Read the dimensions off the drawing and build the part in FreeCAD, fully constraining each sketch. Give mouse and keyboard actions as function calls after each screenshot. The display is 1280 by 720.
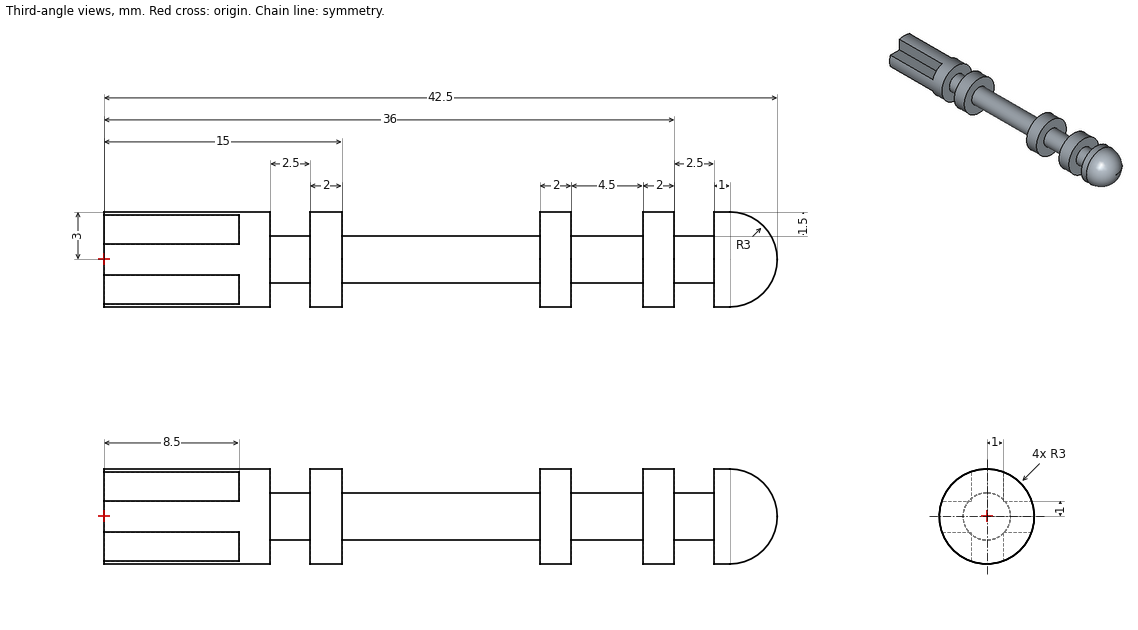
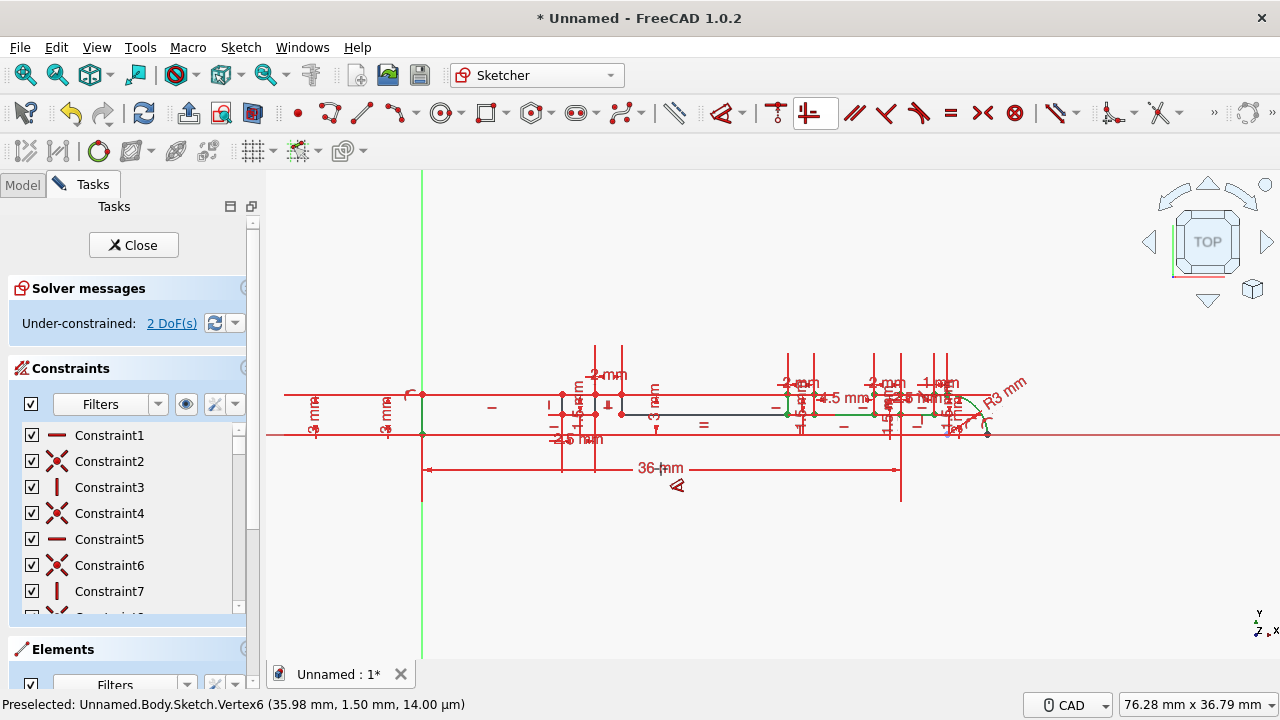
click(622, 415)
click(522, 469)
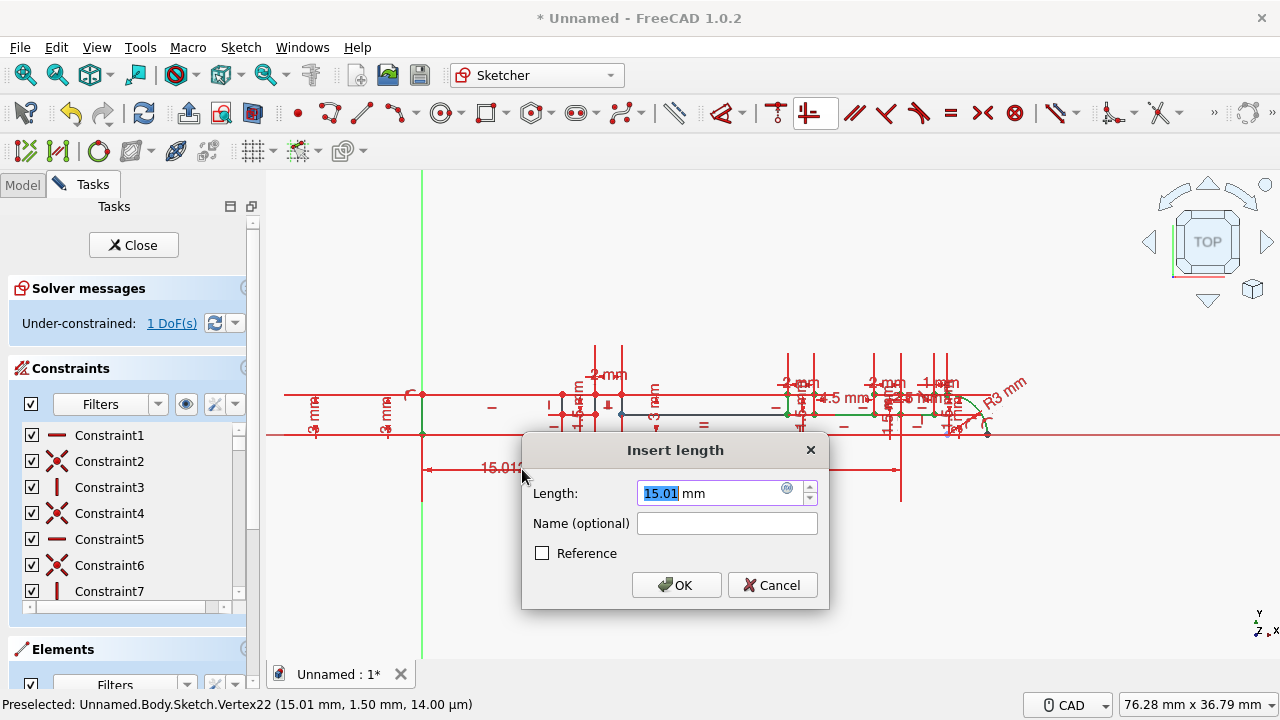
text(15)
key(Return)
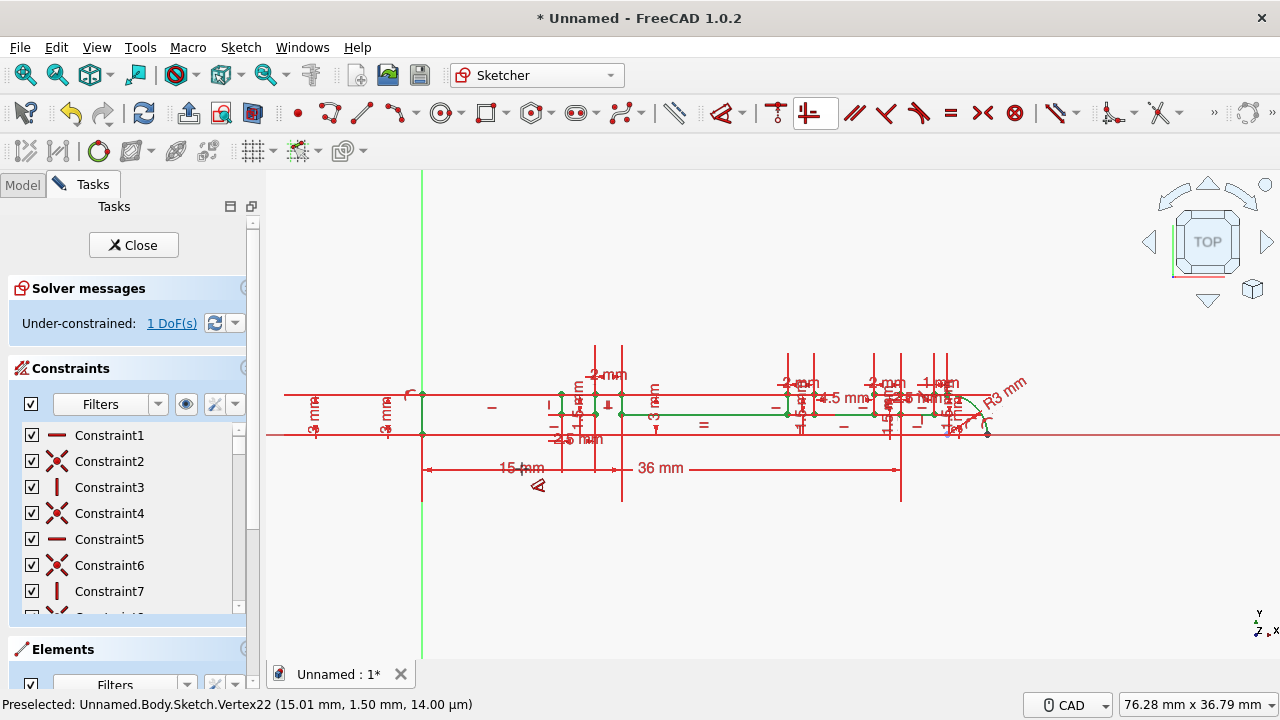
click(592, 435)
click(835, 469)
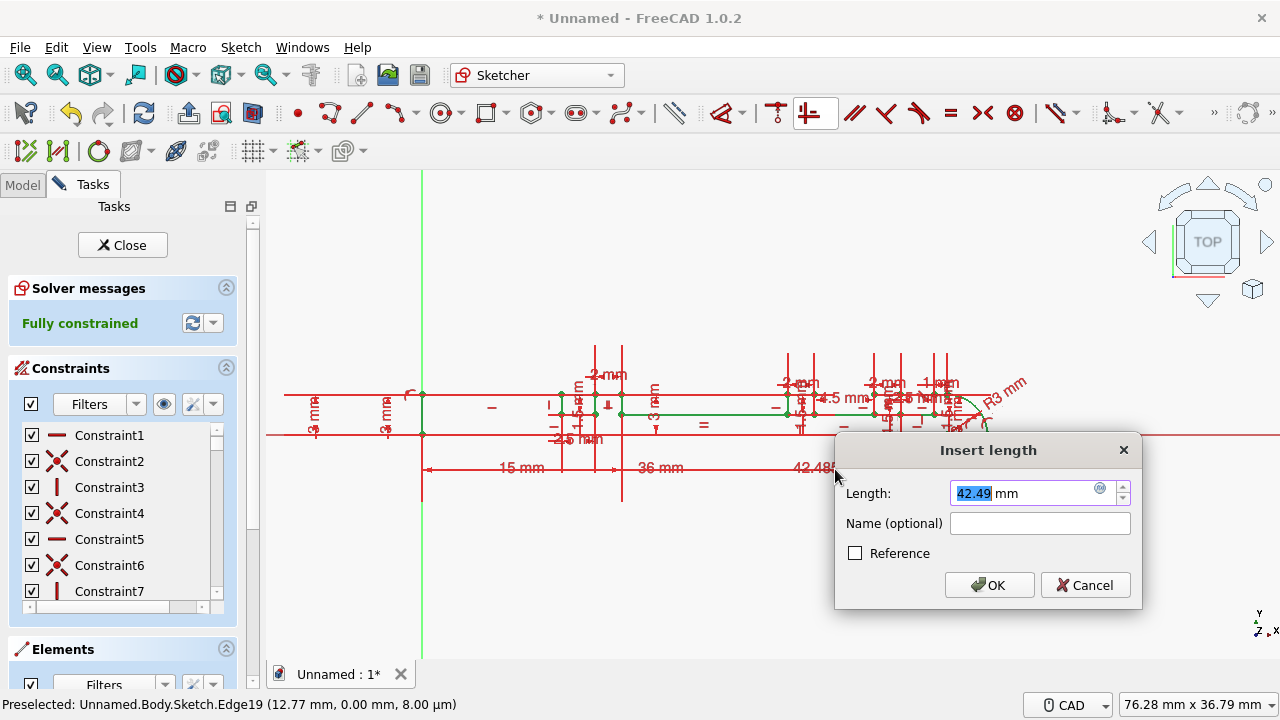
text(42.5)
key(Return)
key(Escape)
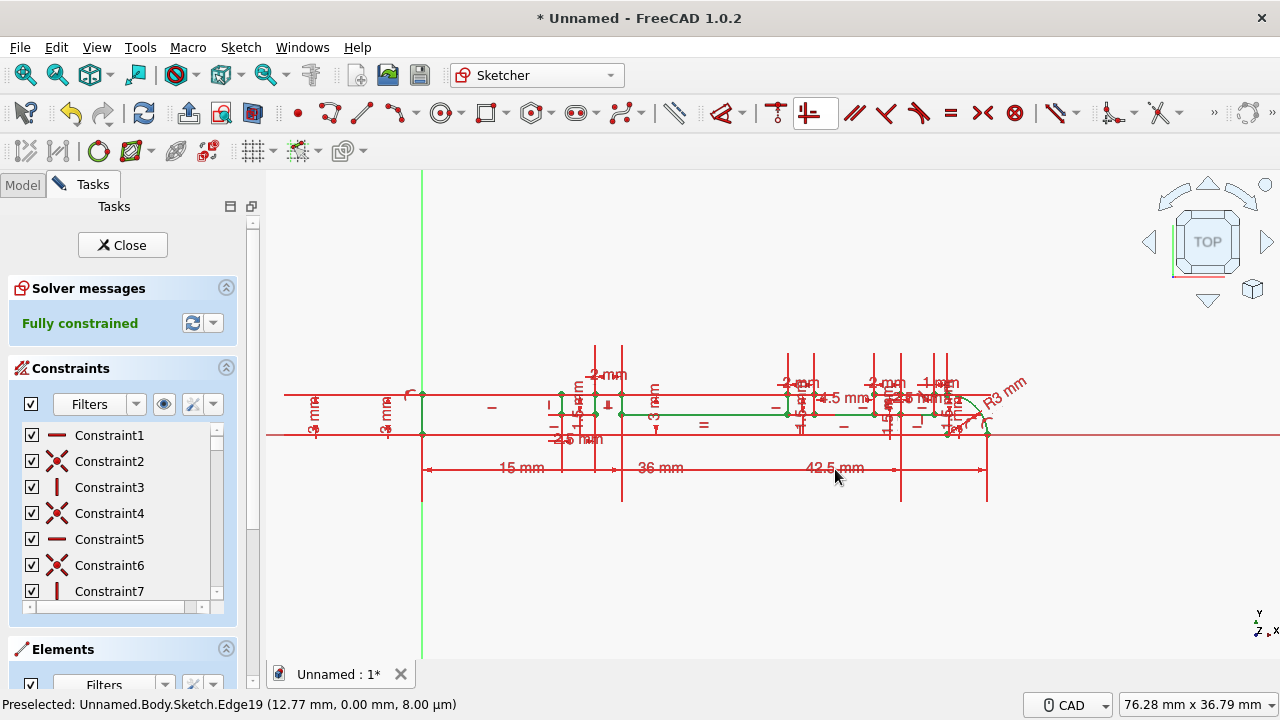
click(123, 245)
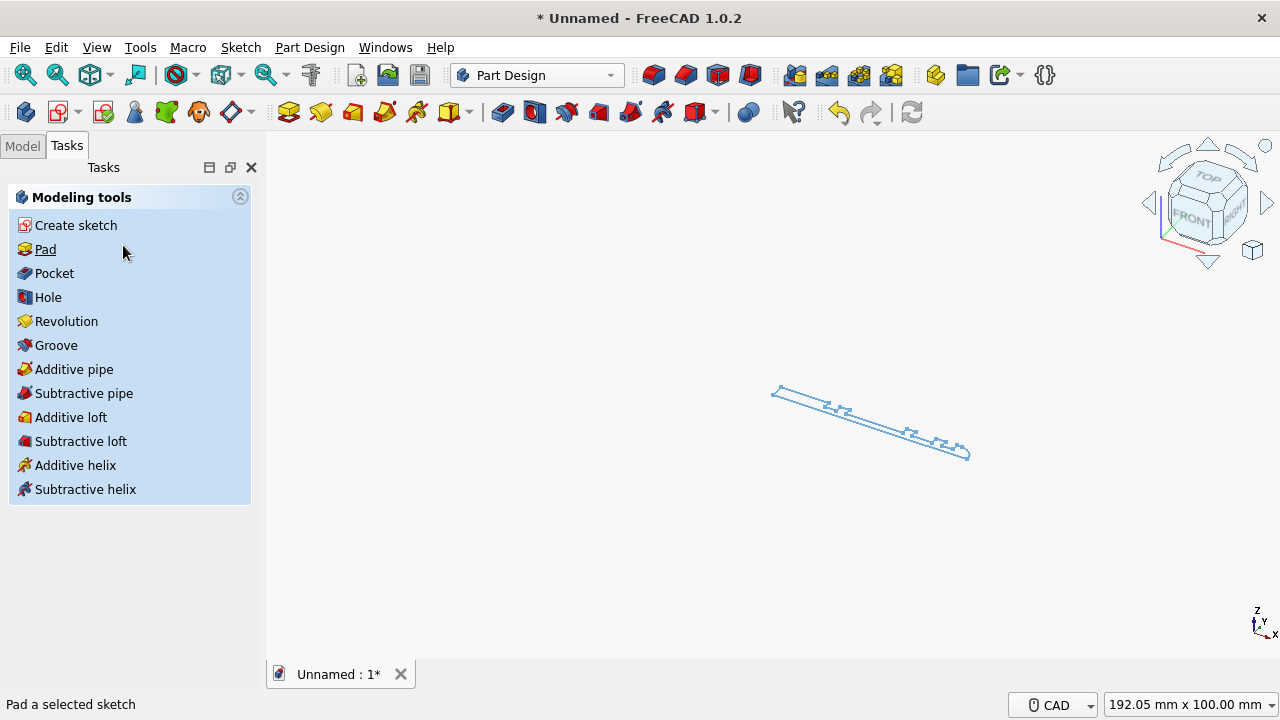
click(322, 112)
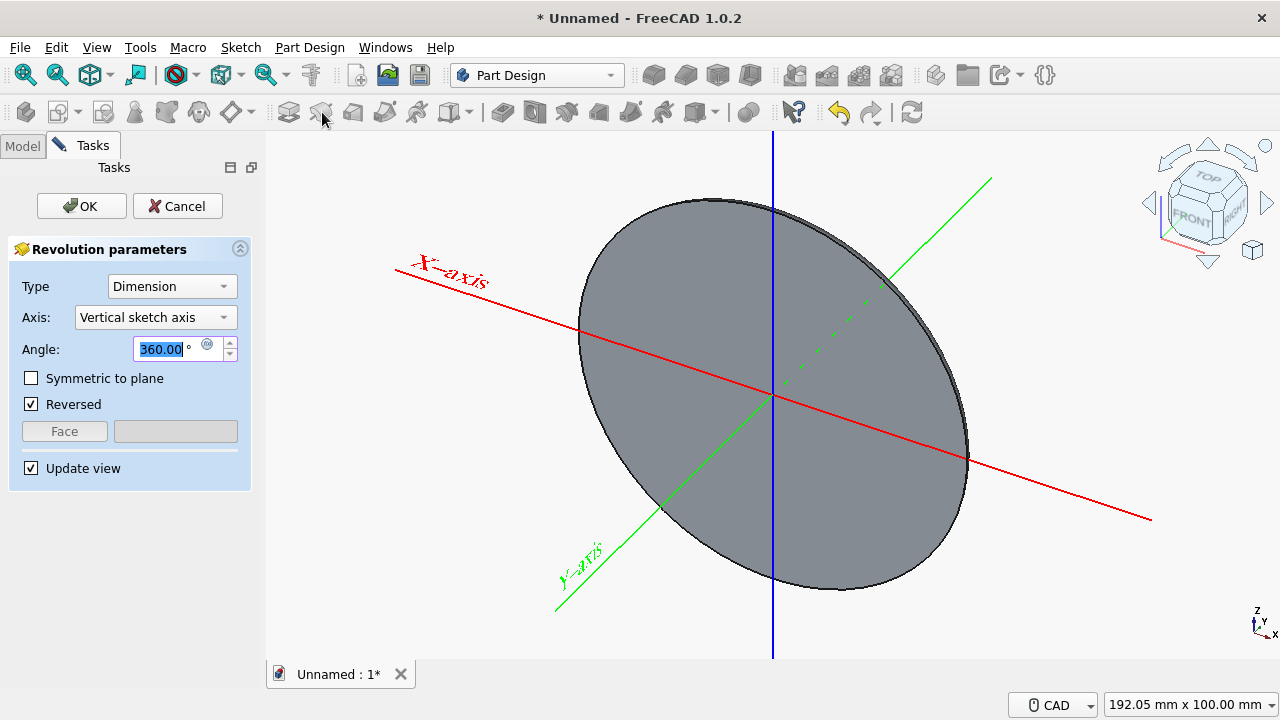
click(156, 318)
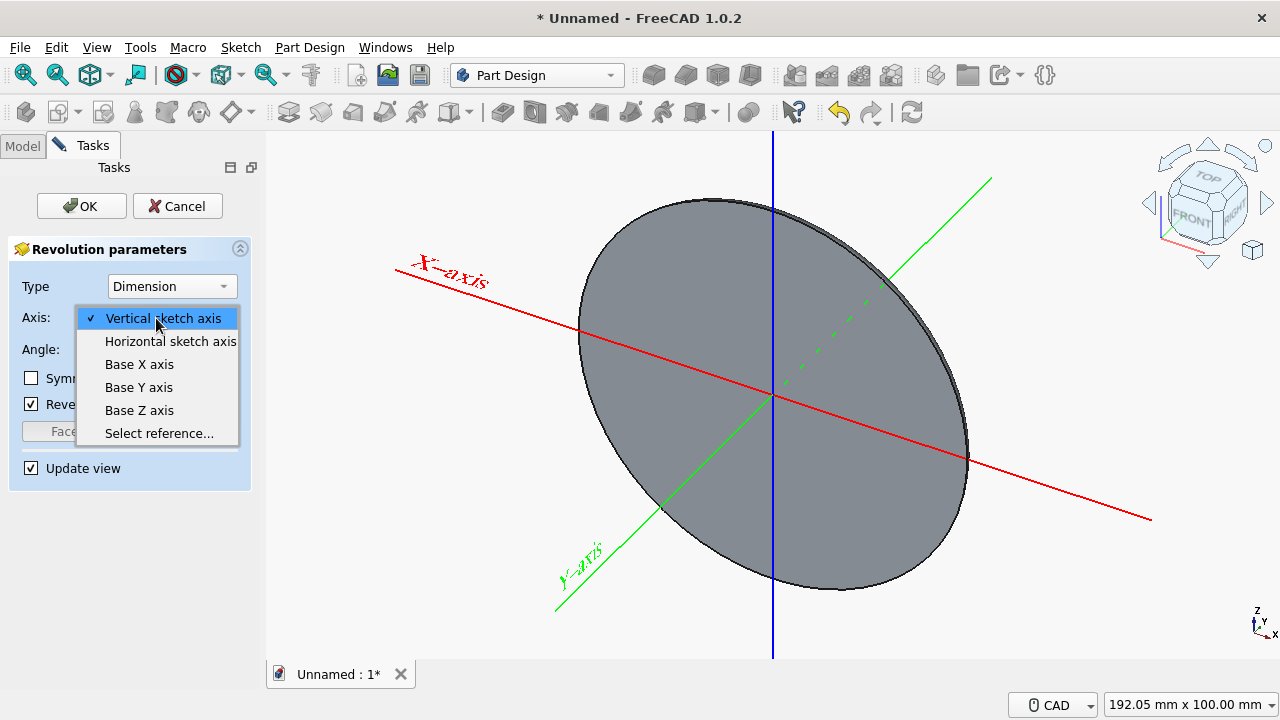
click(156, 342)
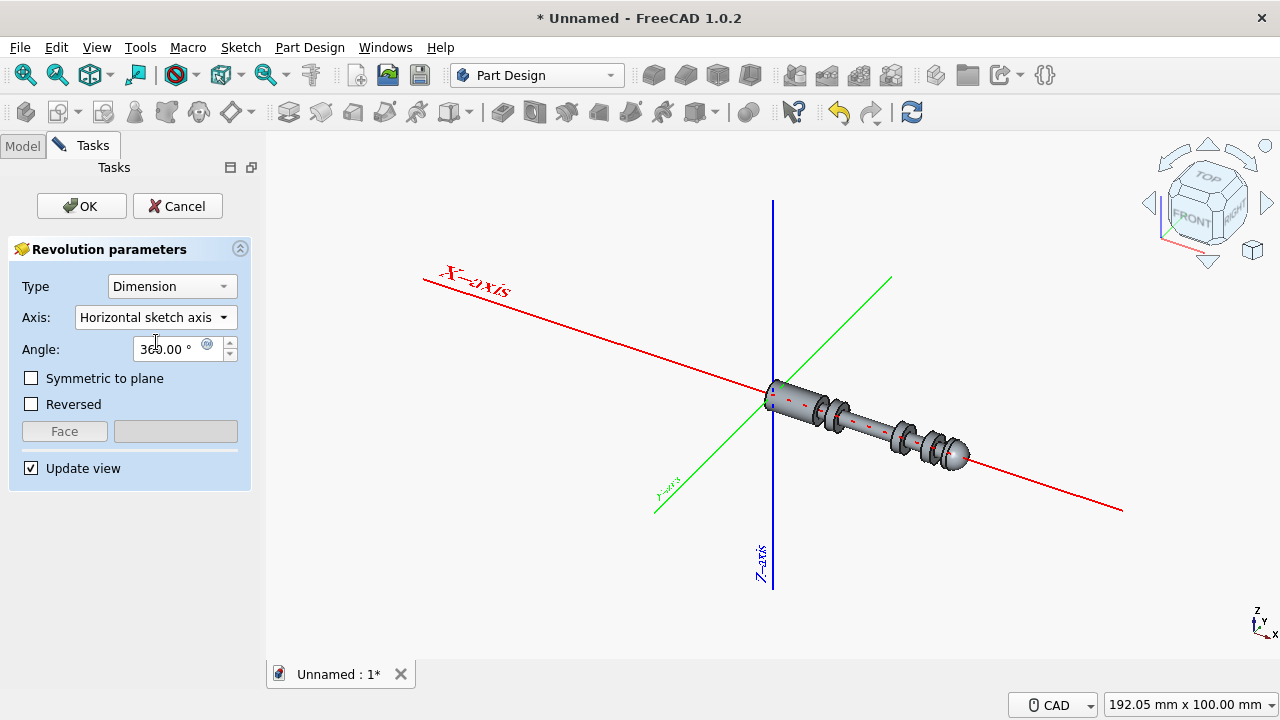
click(82, 206)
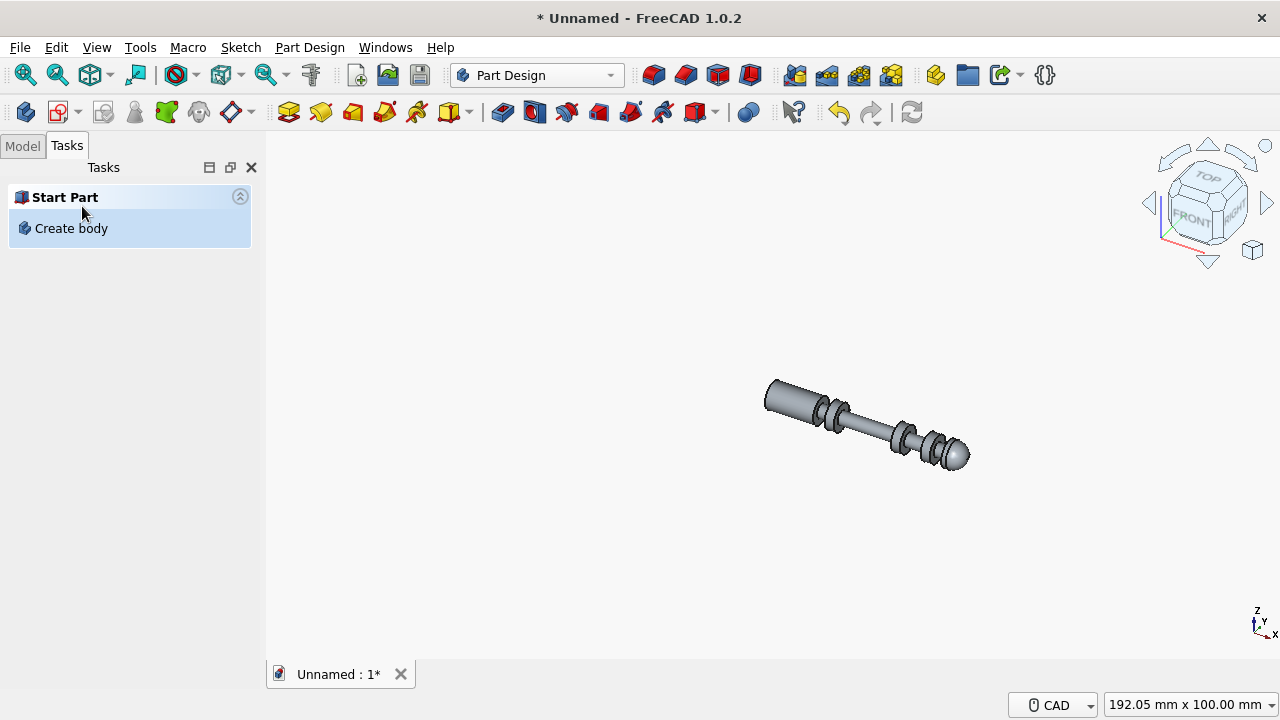
click(26, 76)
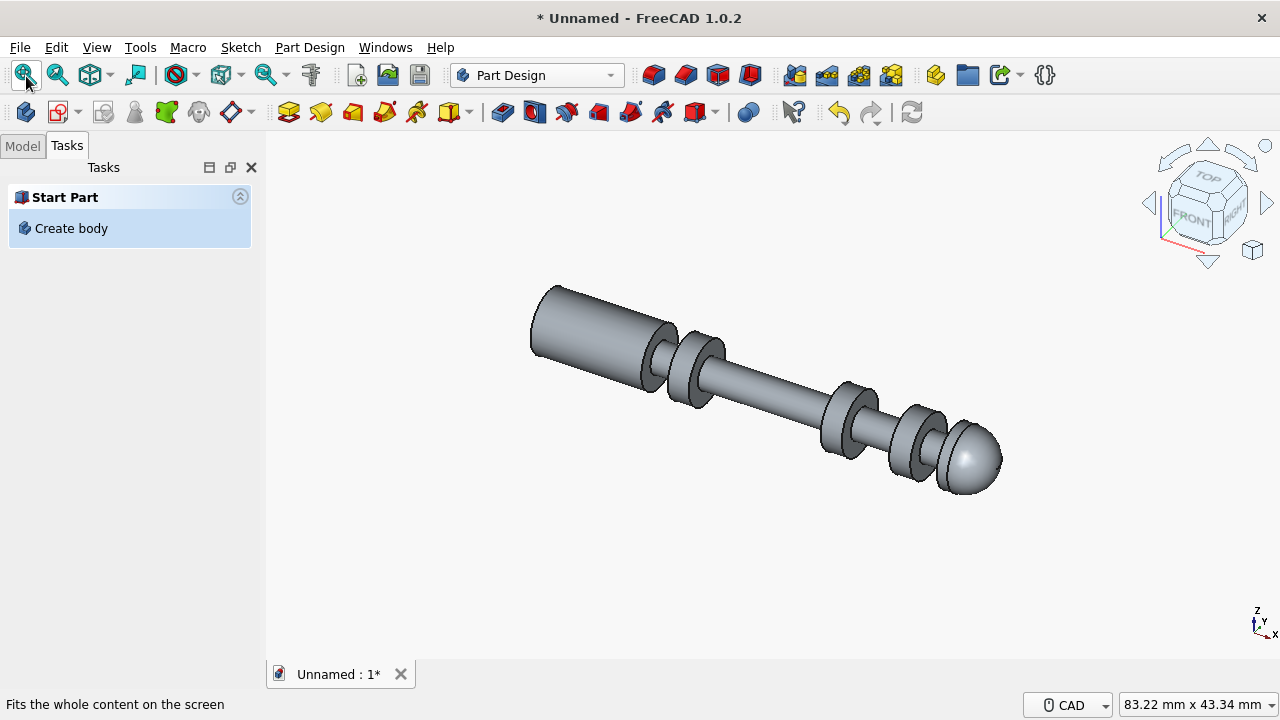
click(23, 145)